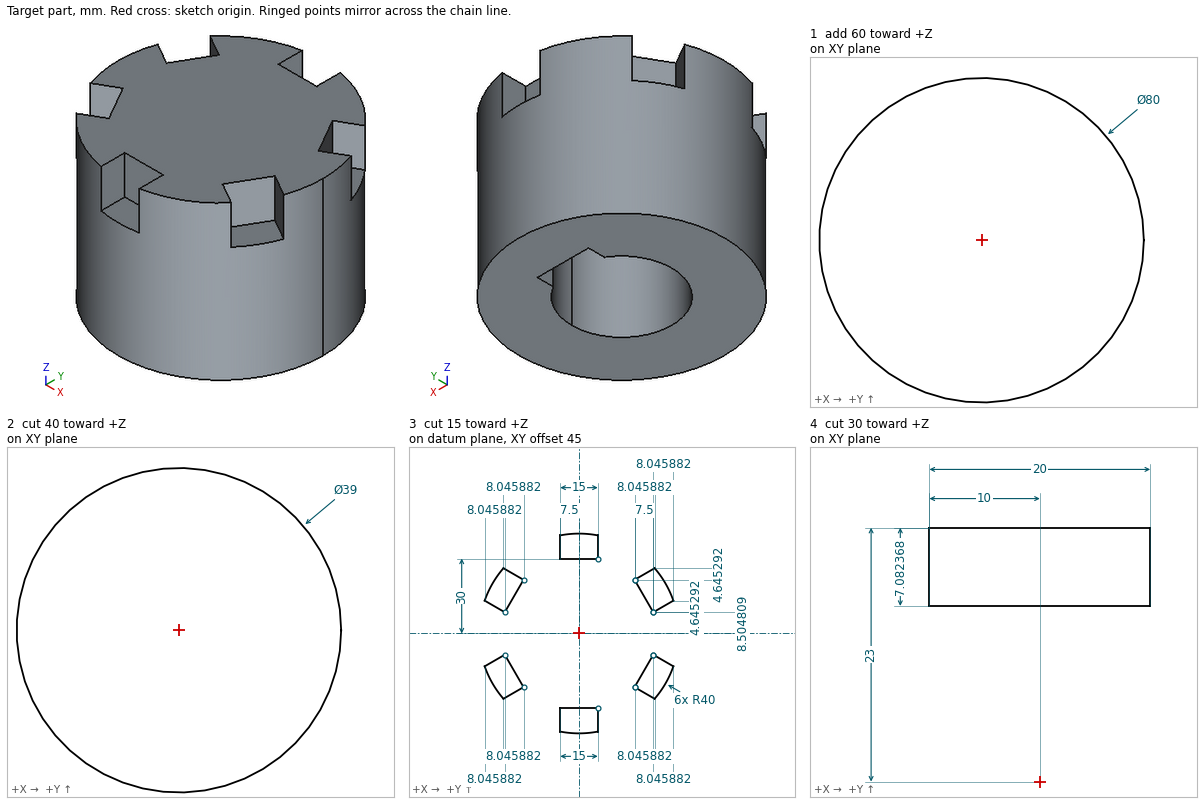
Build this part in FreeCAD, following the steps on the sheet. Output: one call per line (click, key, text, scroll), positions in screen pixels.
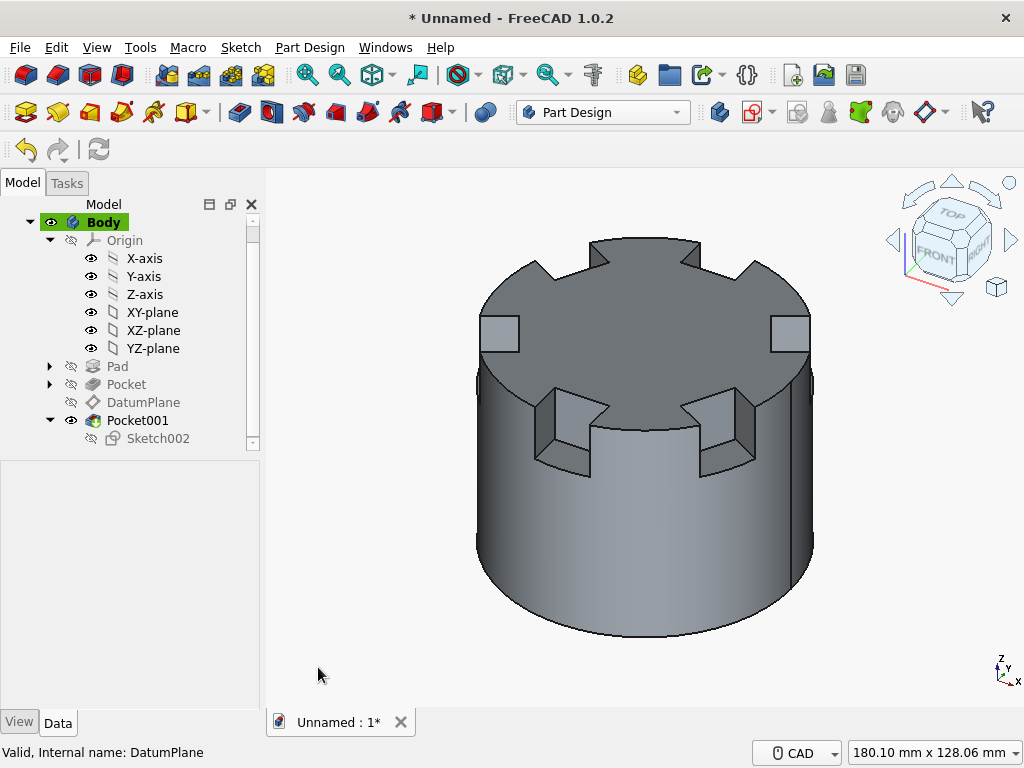
click(752, 112)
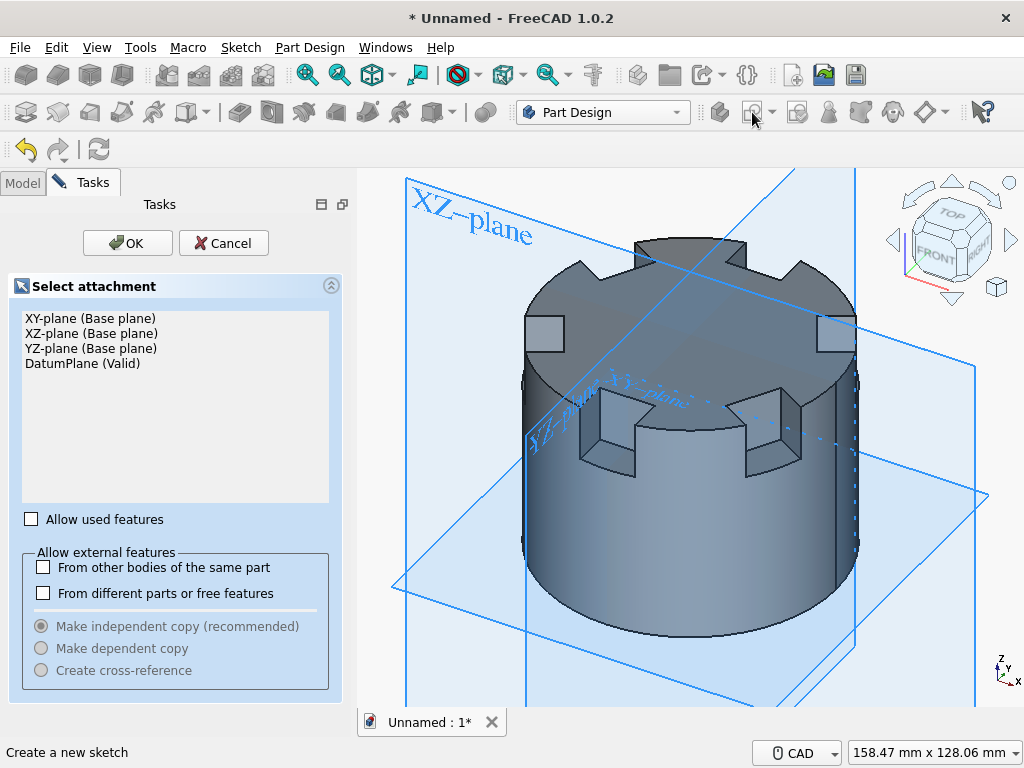
click(82, 318)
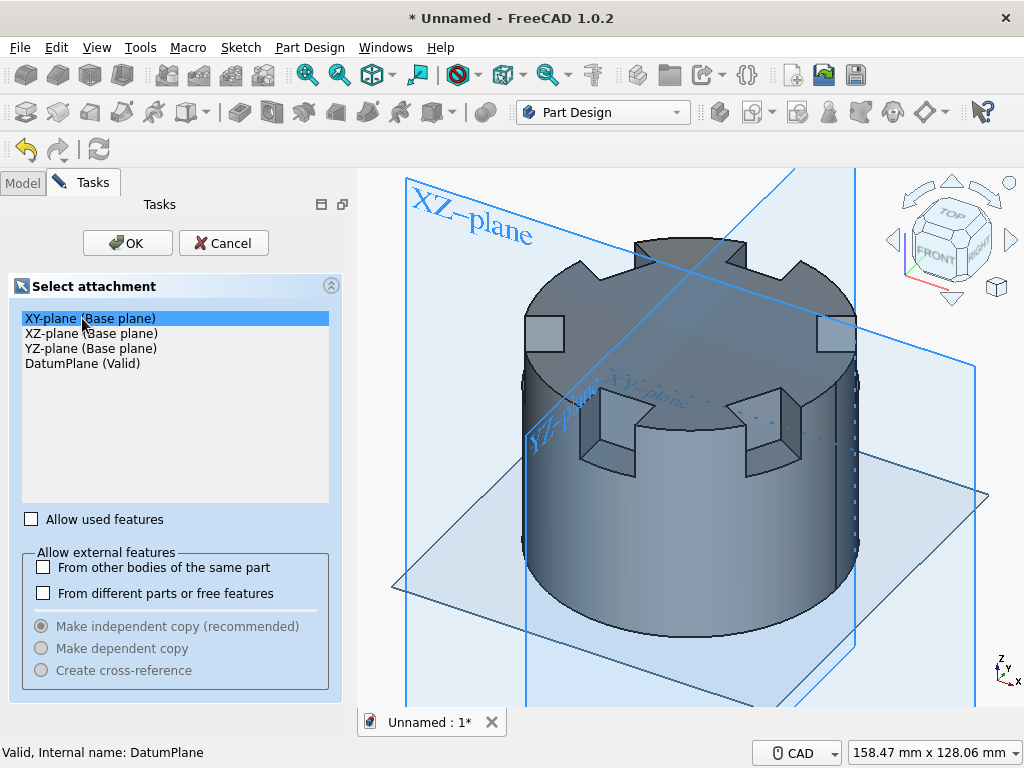
click(128, 243)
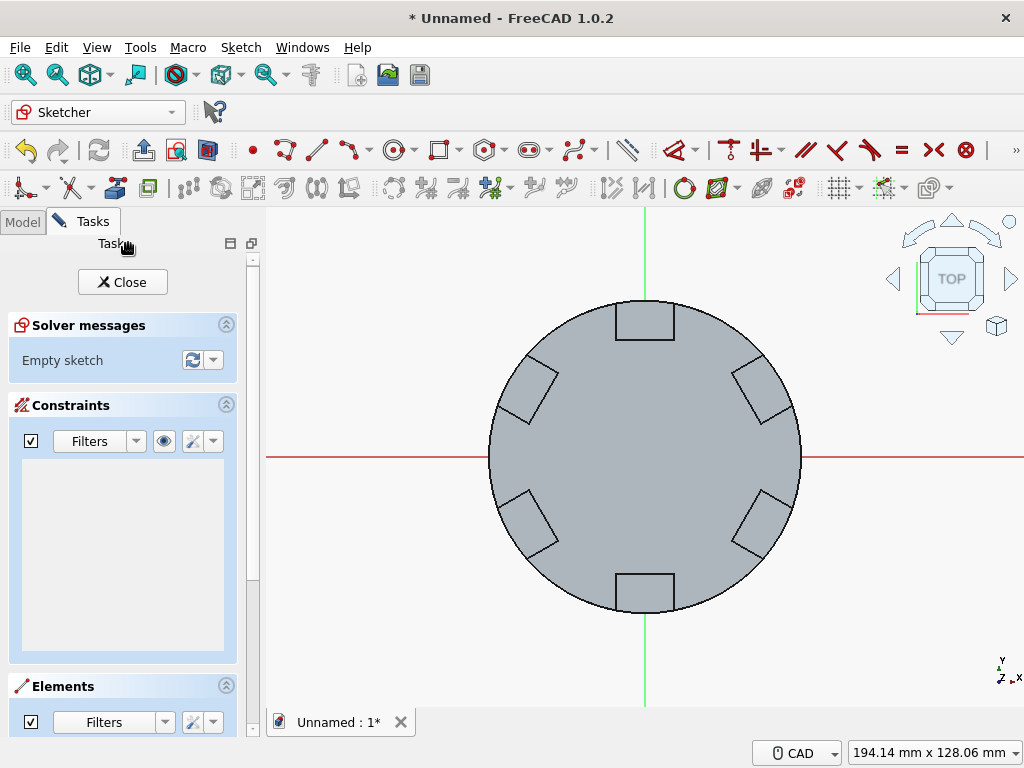
click(208, 150)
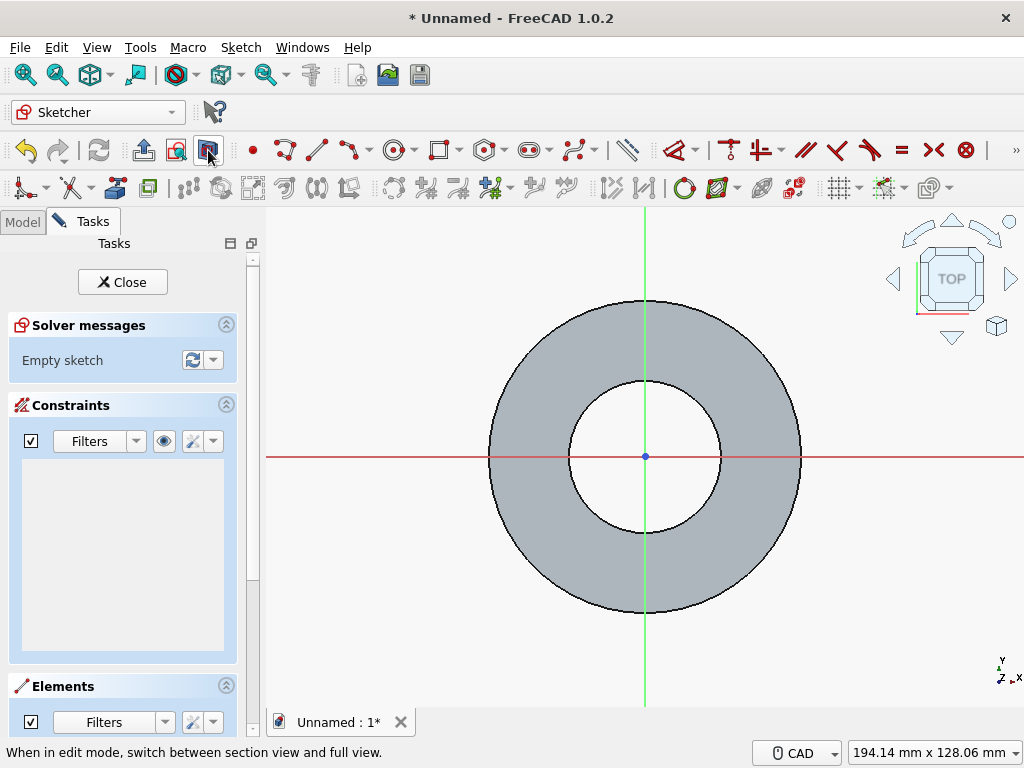
scroll(675, 393, up, 6)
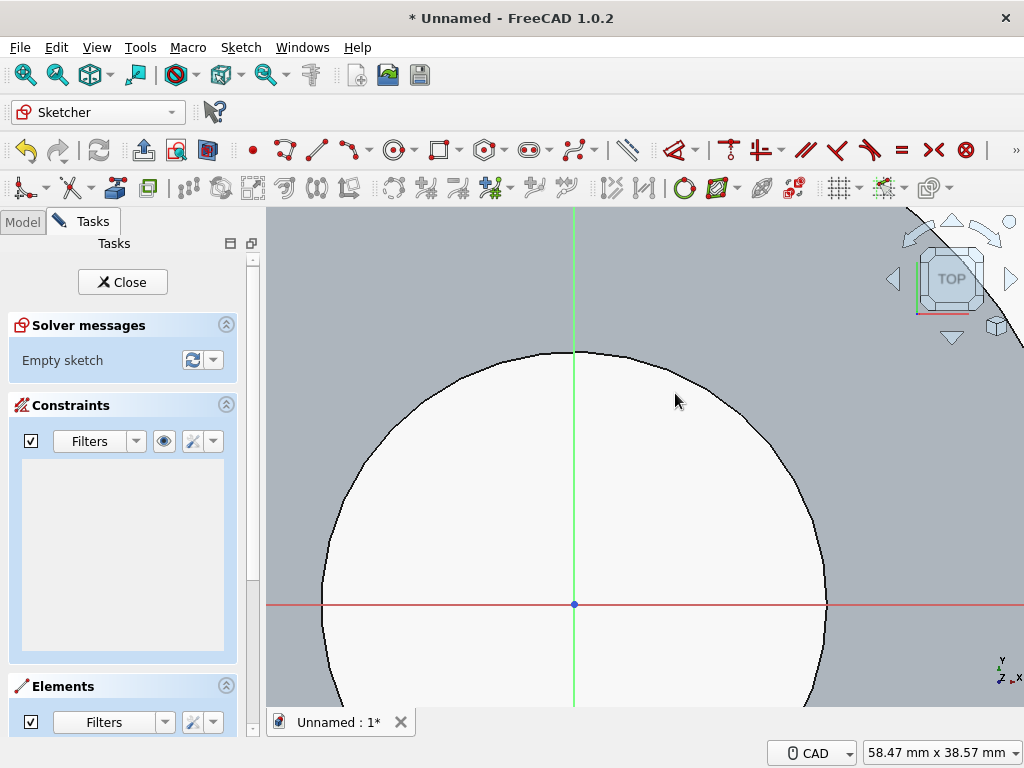
click(440, 150)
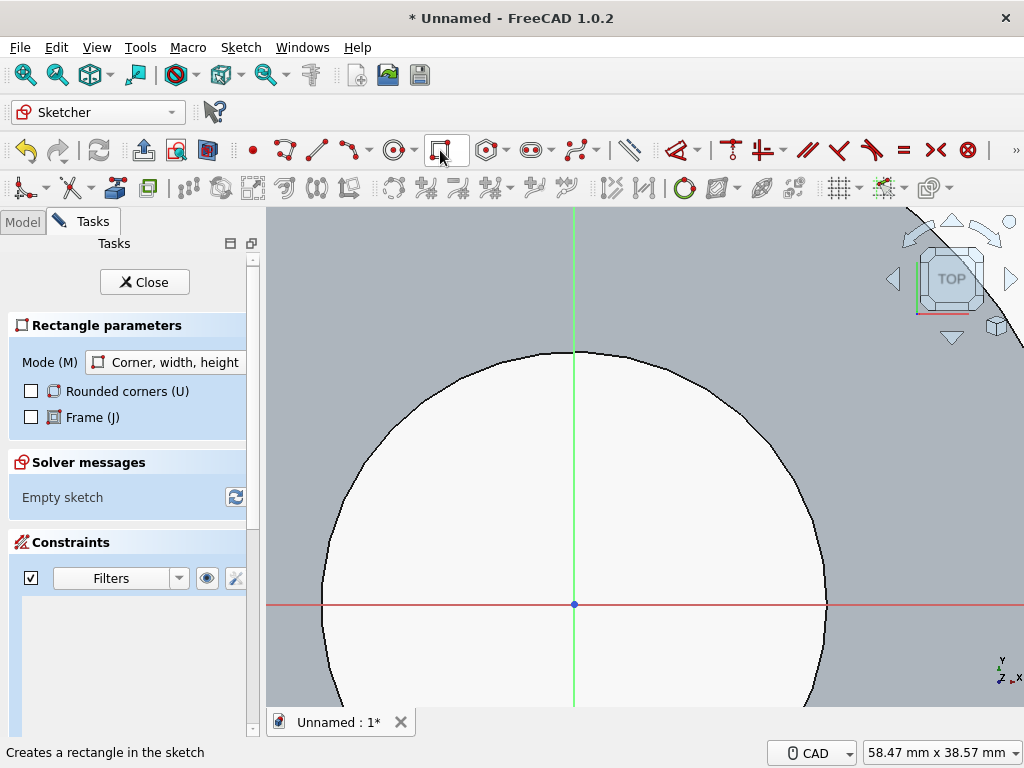
click(445, 306)
click(704, 398)
key(Escape)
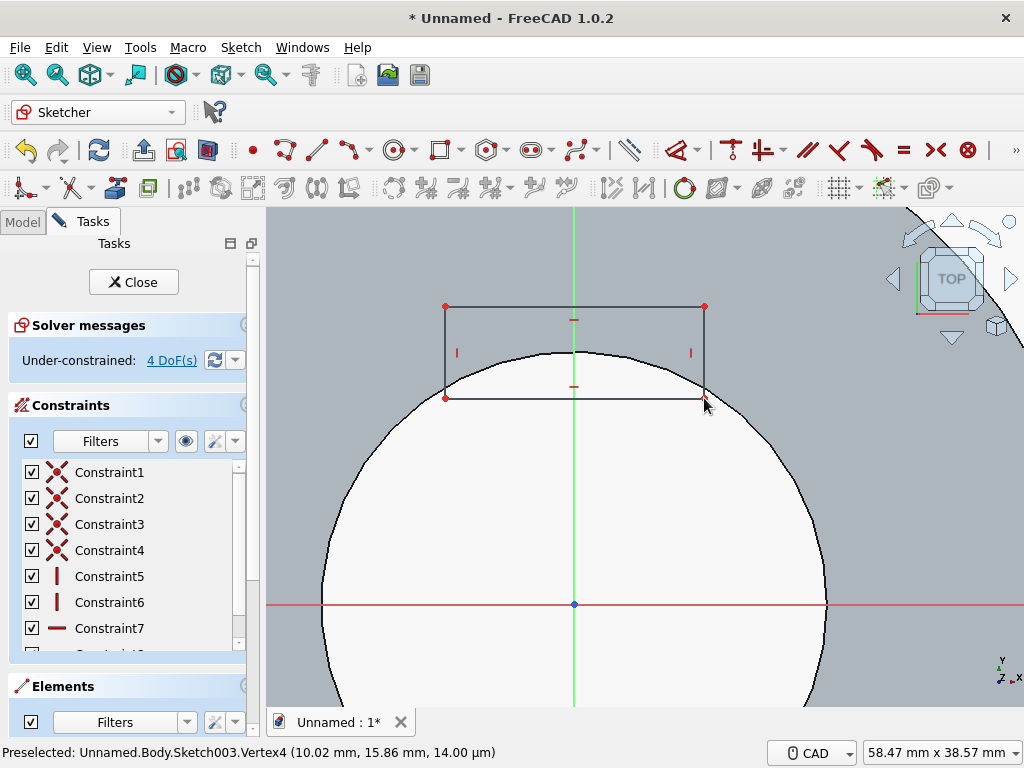
click(676, 150)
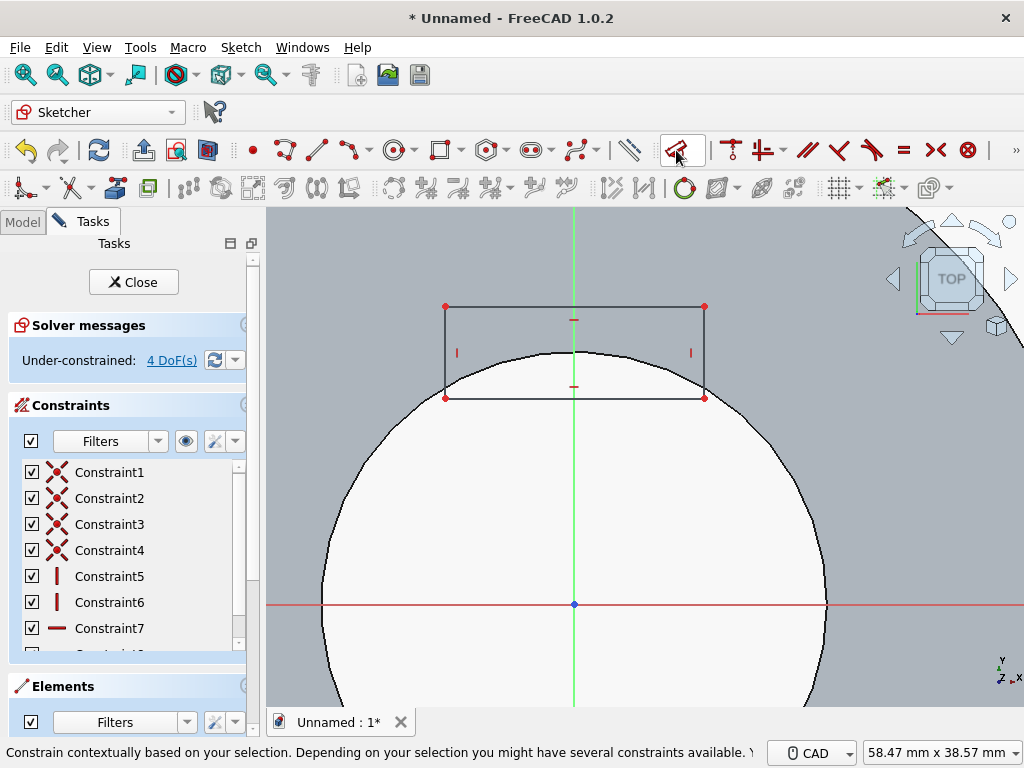
click(523, 399)
click(515, 365)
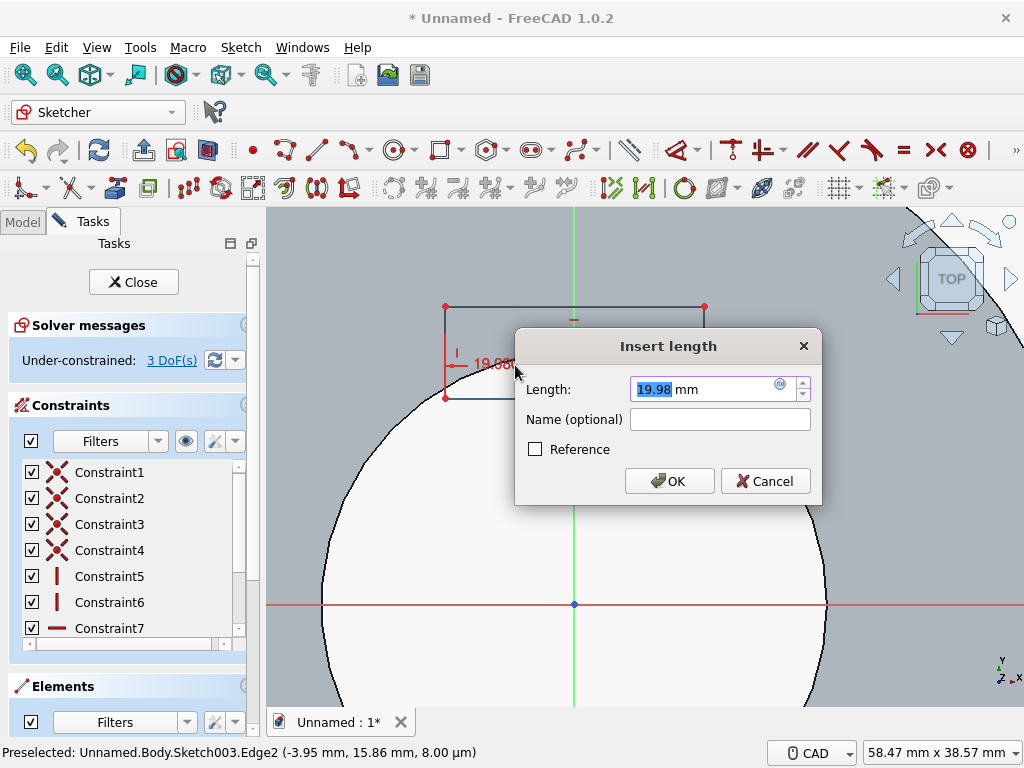
text(20)
key(Return)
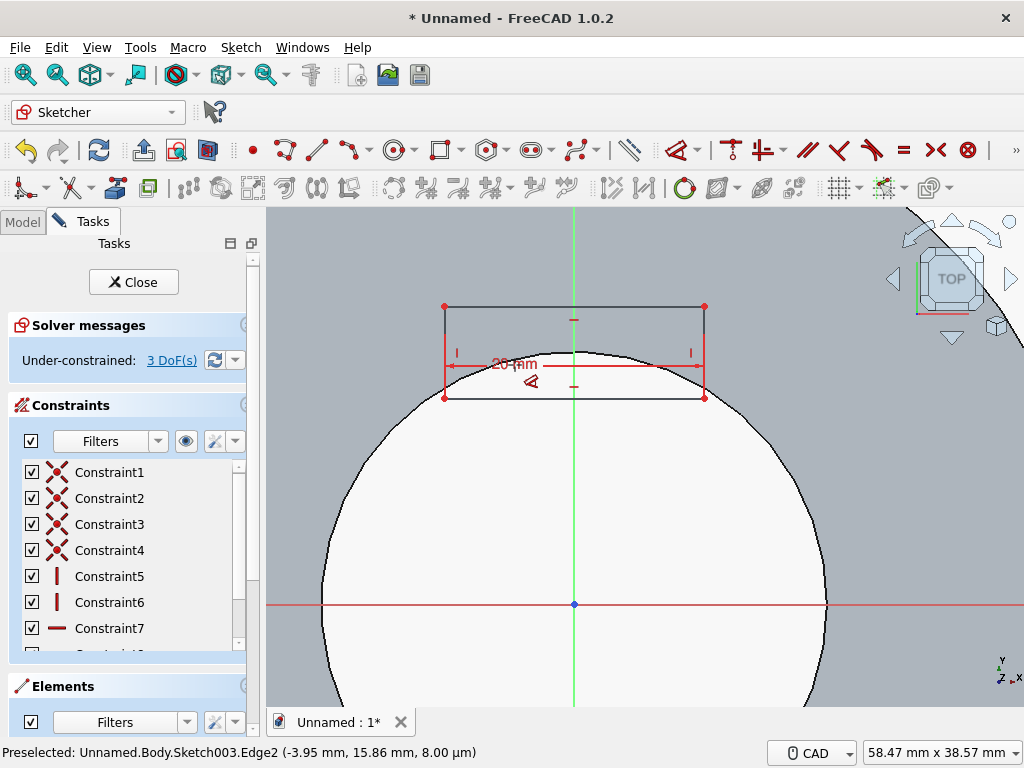
click(445, 307)
click(509, 639)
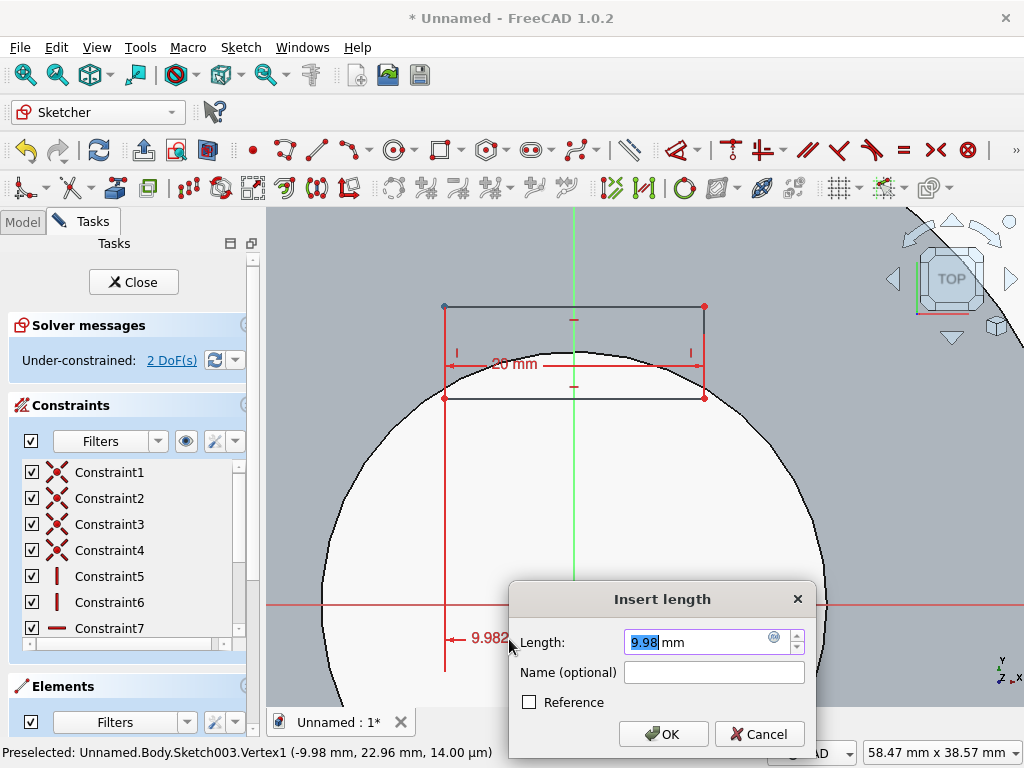
text(10)
key(Return)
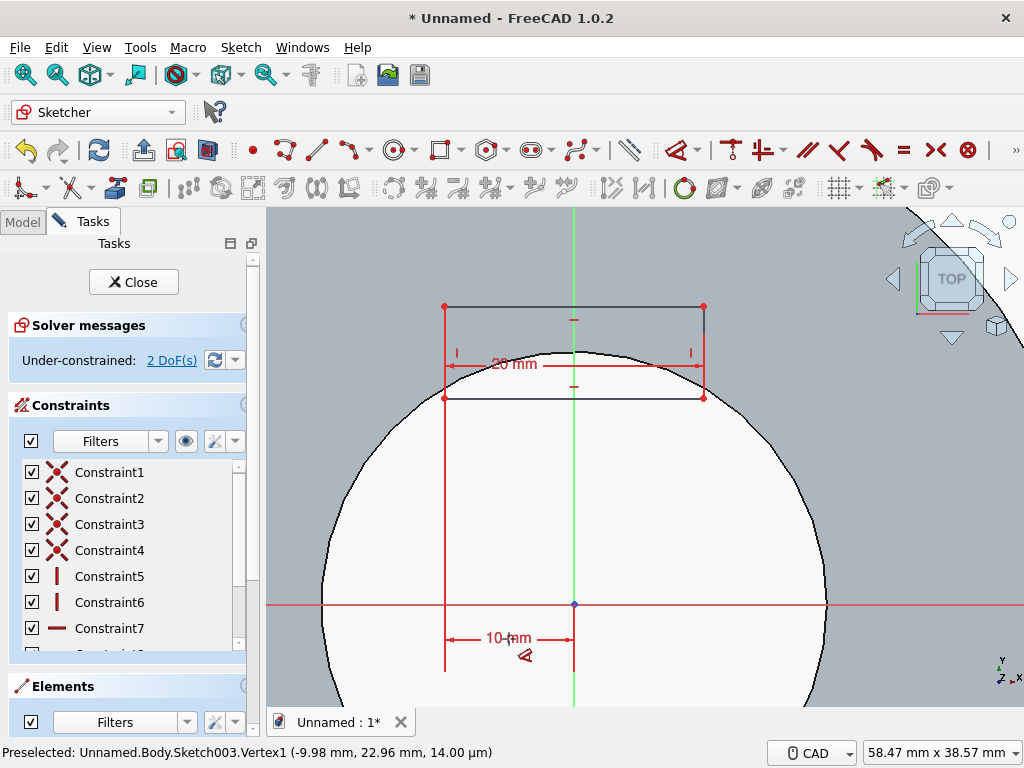
click(445, 307)
click(411, 456)